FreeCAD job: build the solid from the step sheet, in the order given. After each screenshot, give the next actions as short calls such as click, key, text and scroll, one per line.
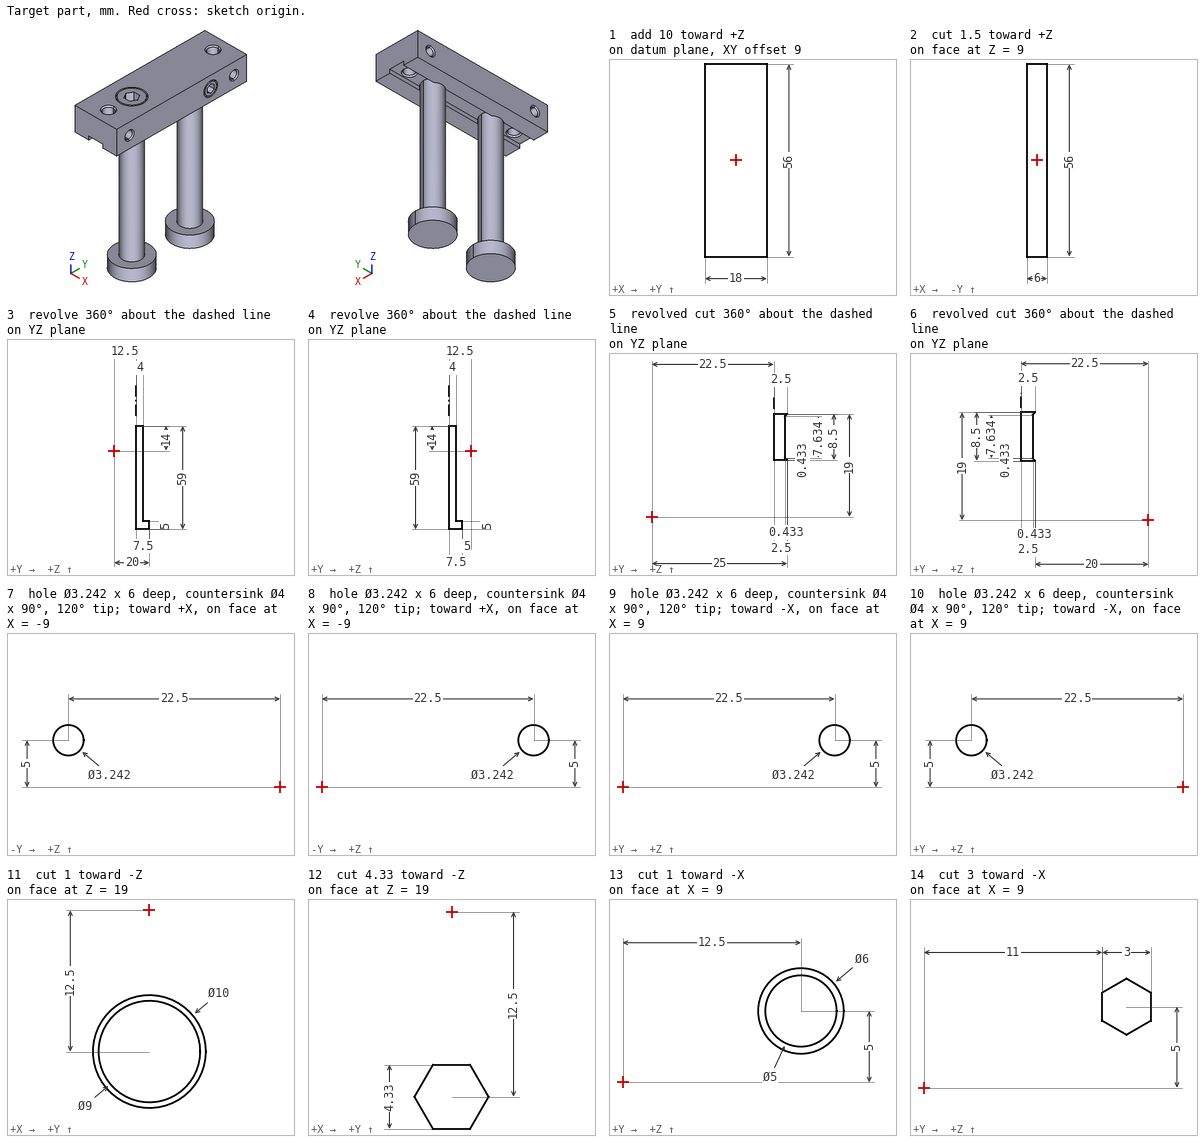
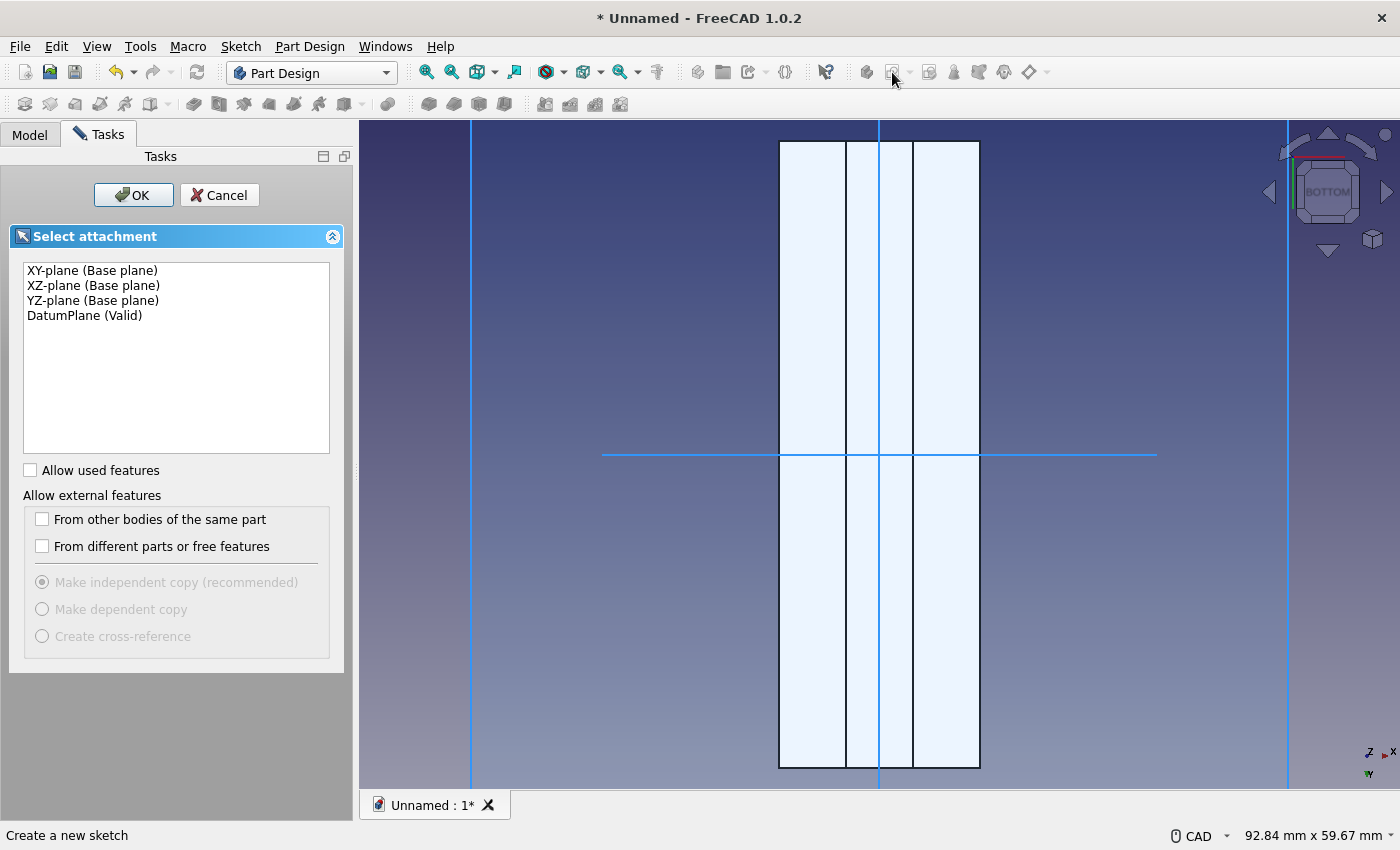
click(84, 300)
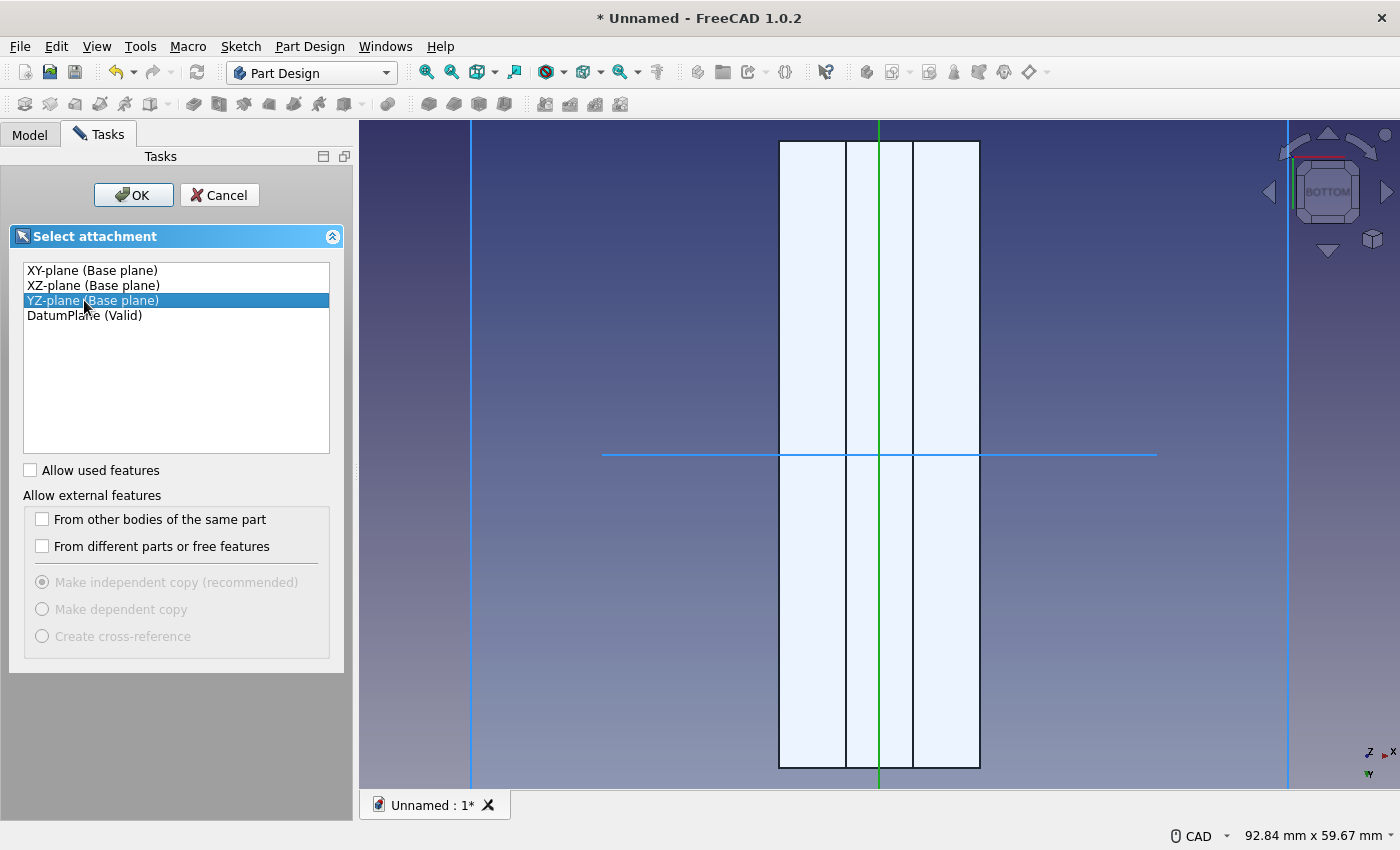
click(134, 195)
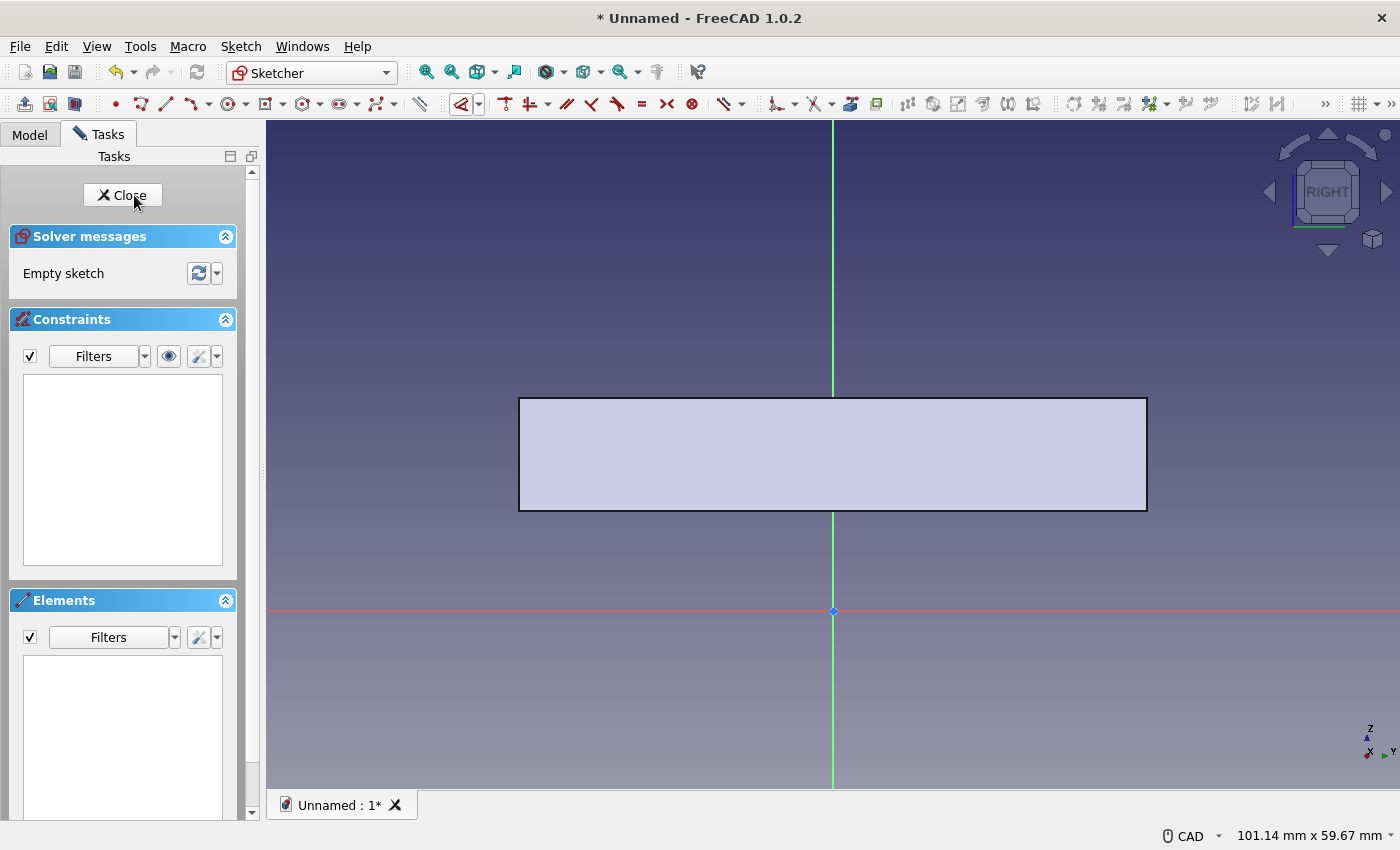
click(75, 104)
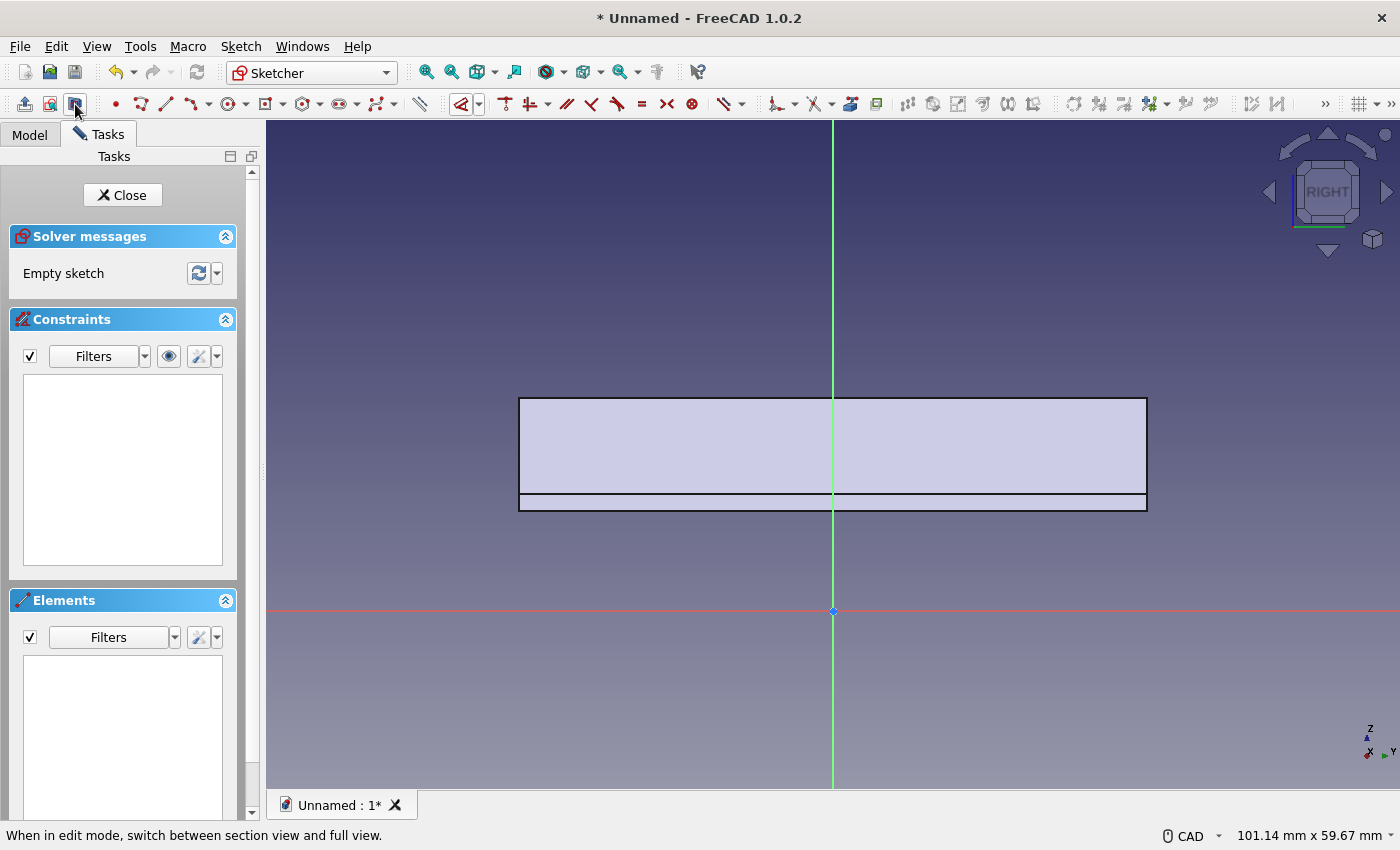
scroll(617, 293, down, 4)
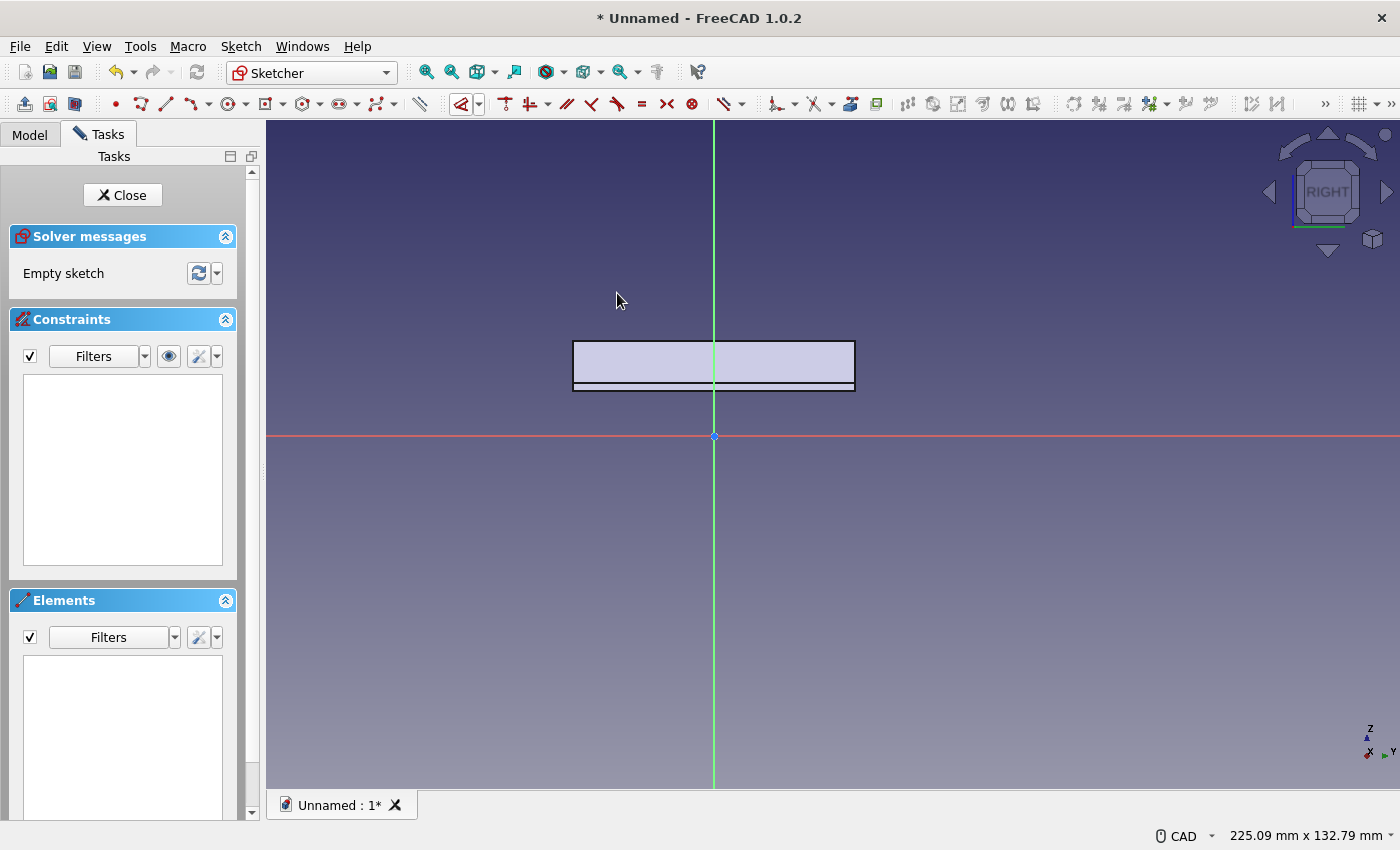
click(141, 104)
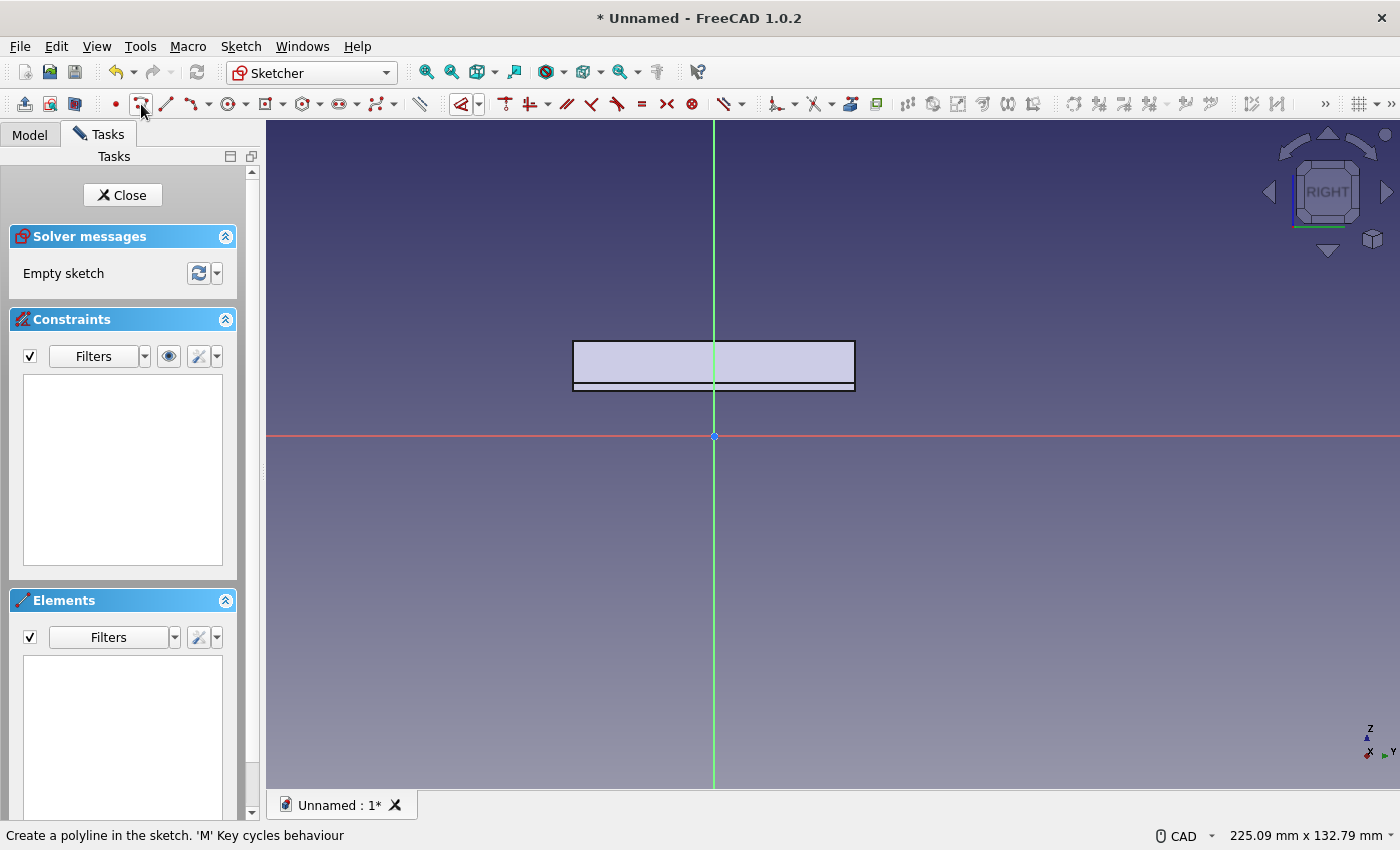
click(777, 366)
click(777, 663)
click(815, 663)
click(815, 638)
click(797, 638)
click(797, 366)
click(777, 367)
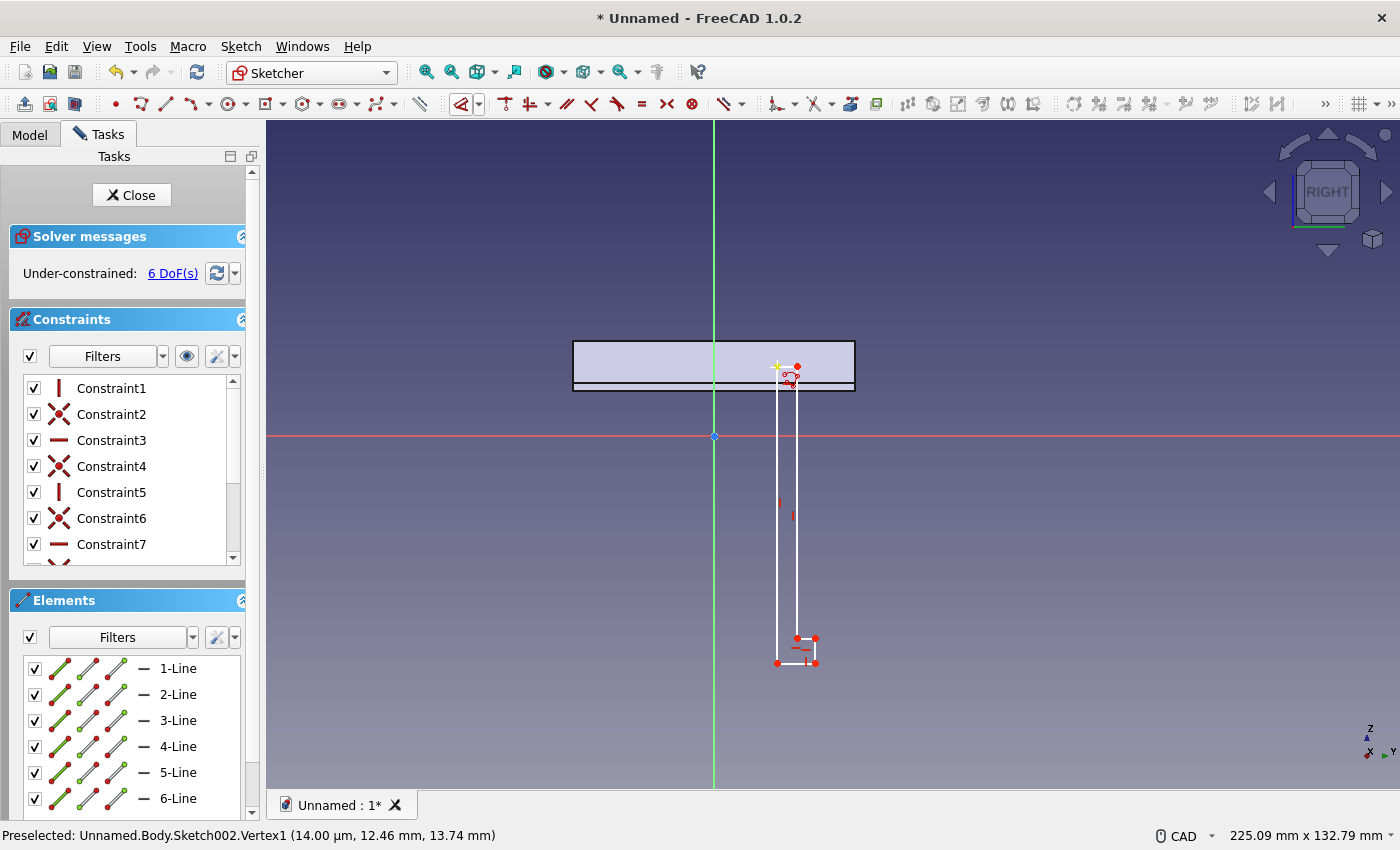
click(166, 104)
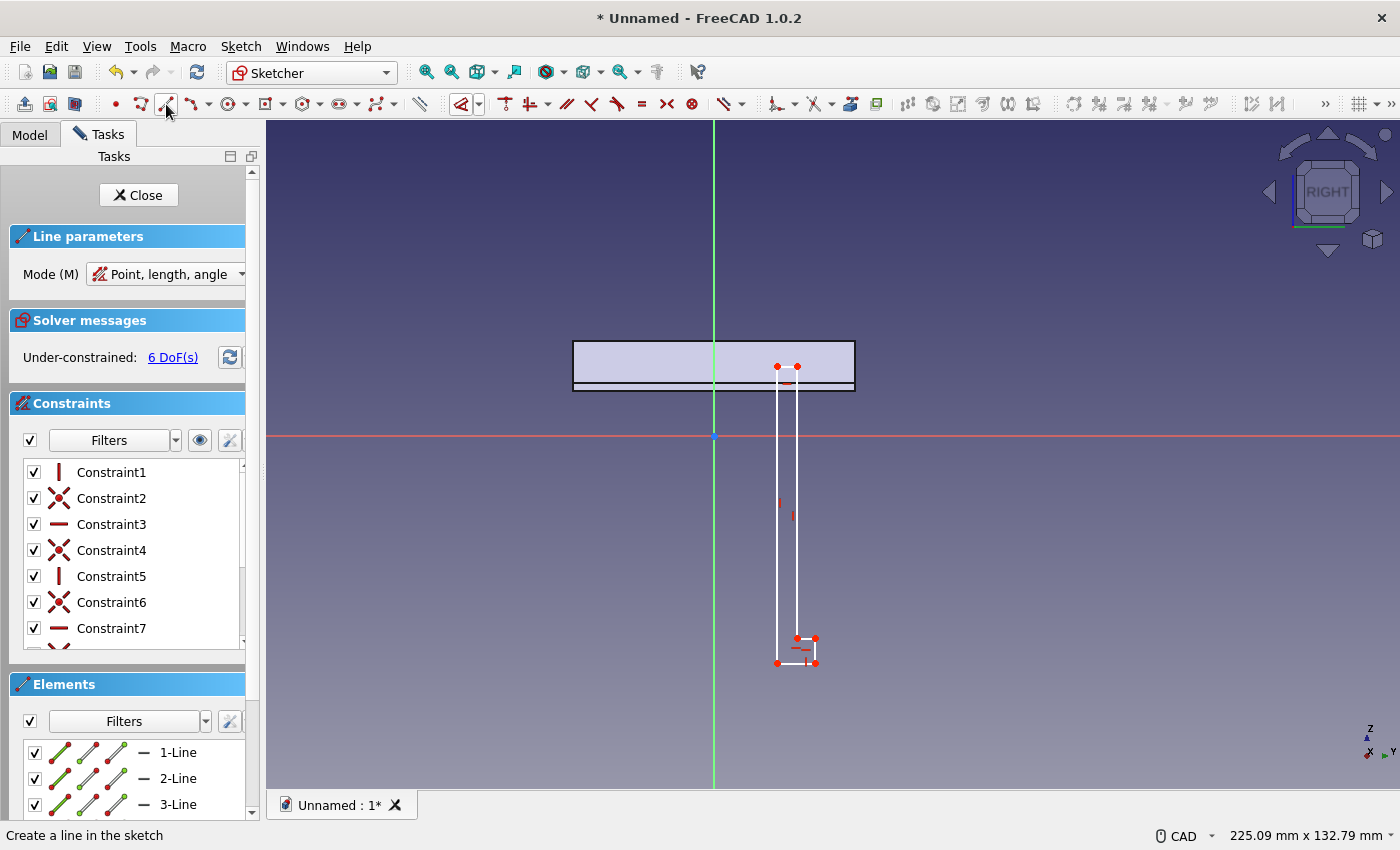
click(777, 336)
click(777, 247)
key(Escape)